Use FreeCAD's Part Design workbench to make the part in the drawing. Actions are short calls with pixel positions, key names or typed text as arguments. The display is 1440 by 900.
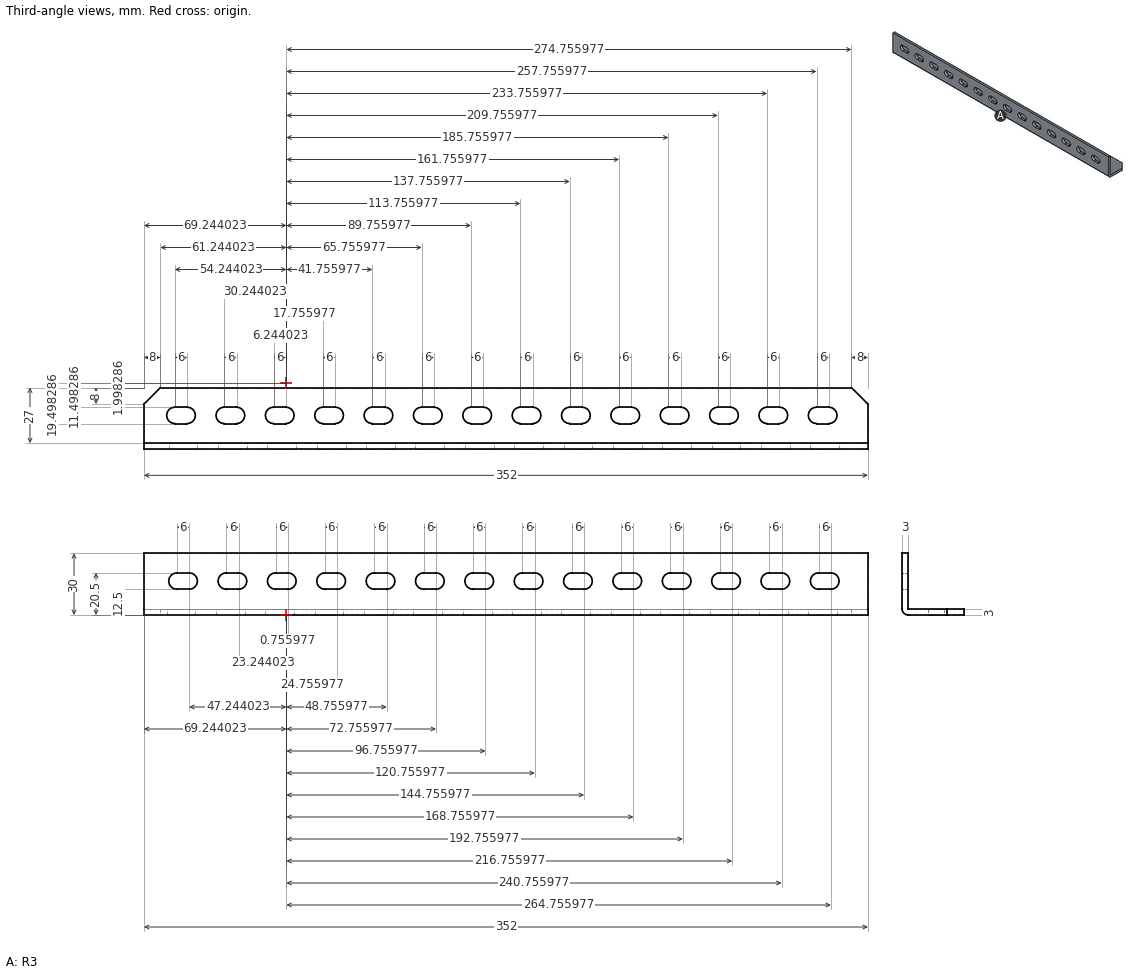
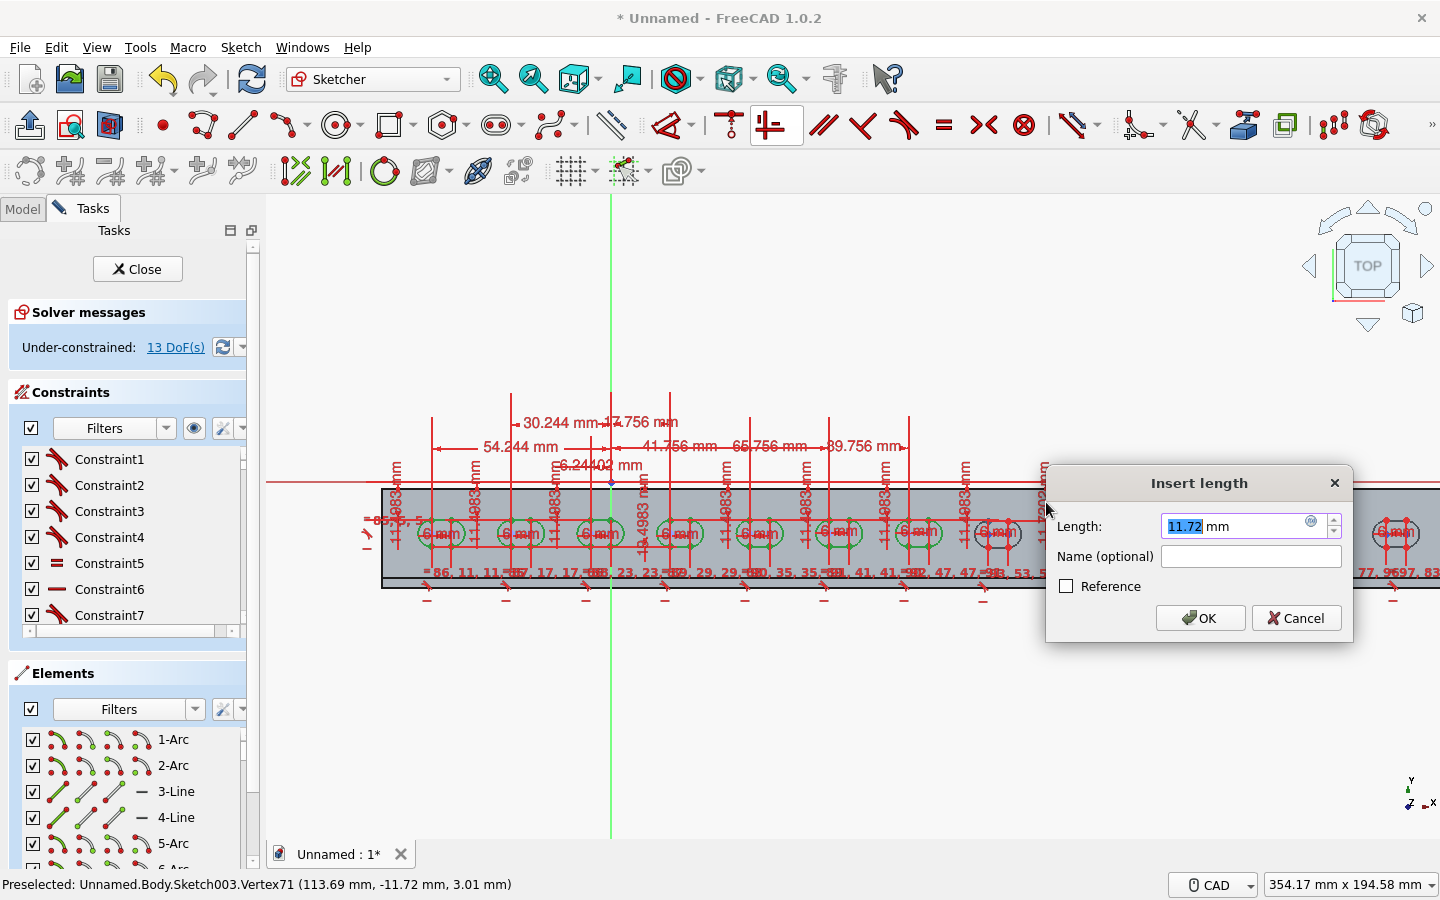
text(11.498286)
key(Return)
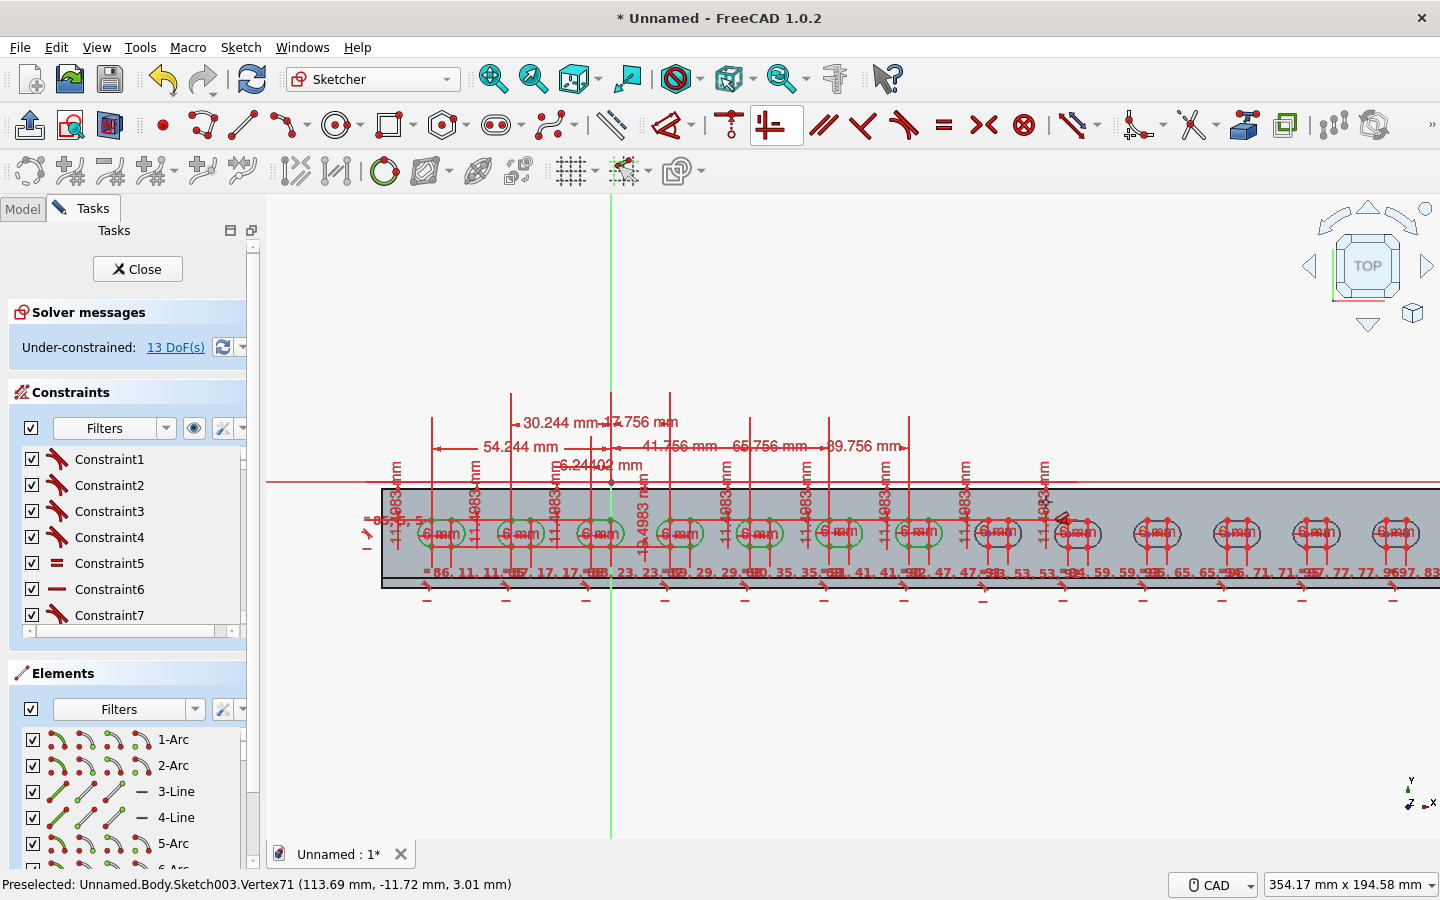
click(1068, 521)
click(1126, 502)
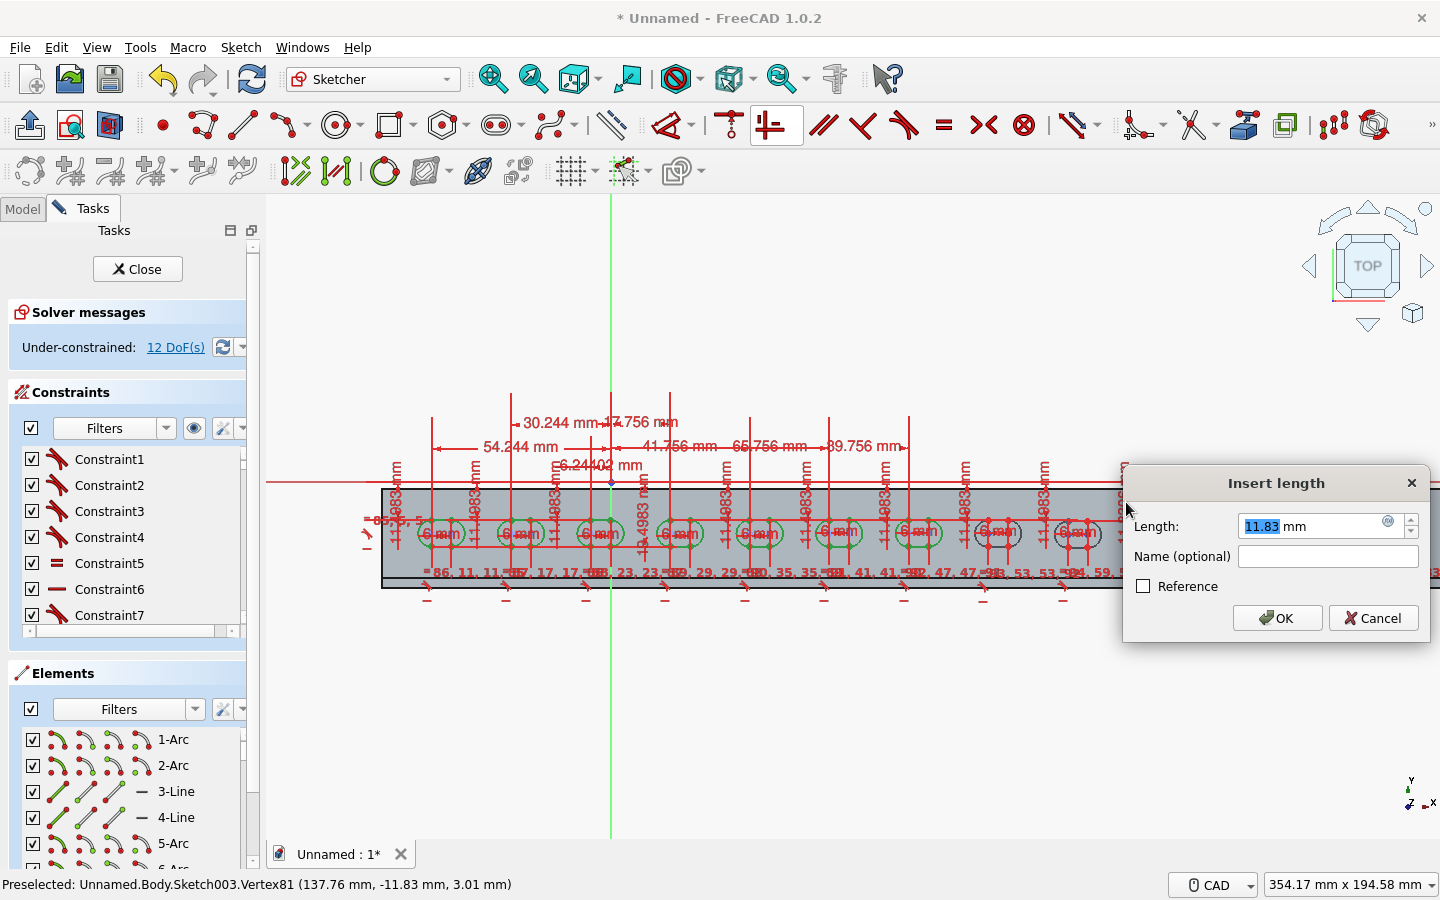
text(11.498286)
key(Return)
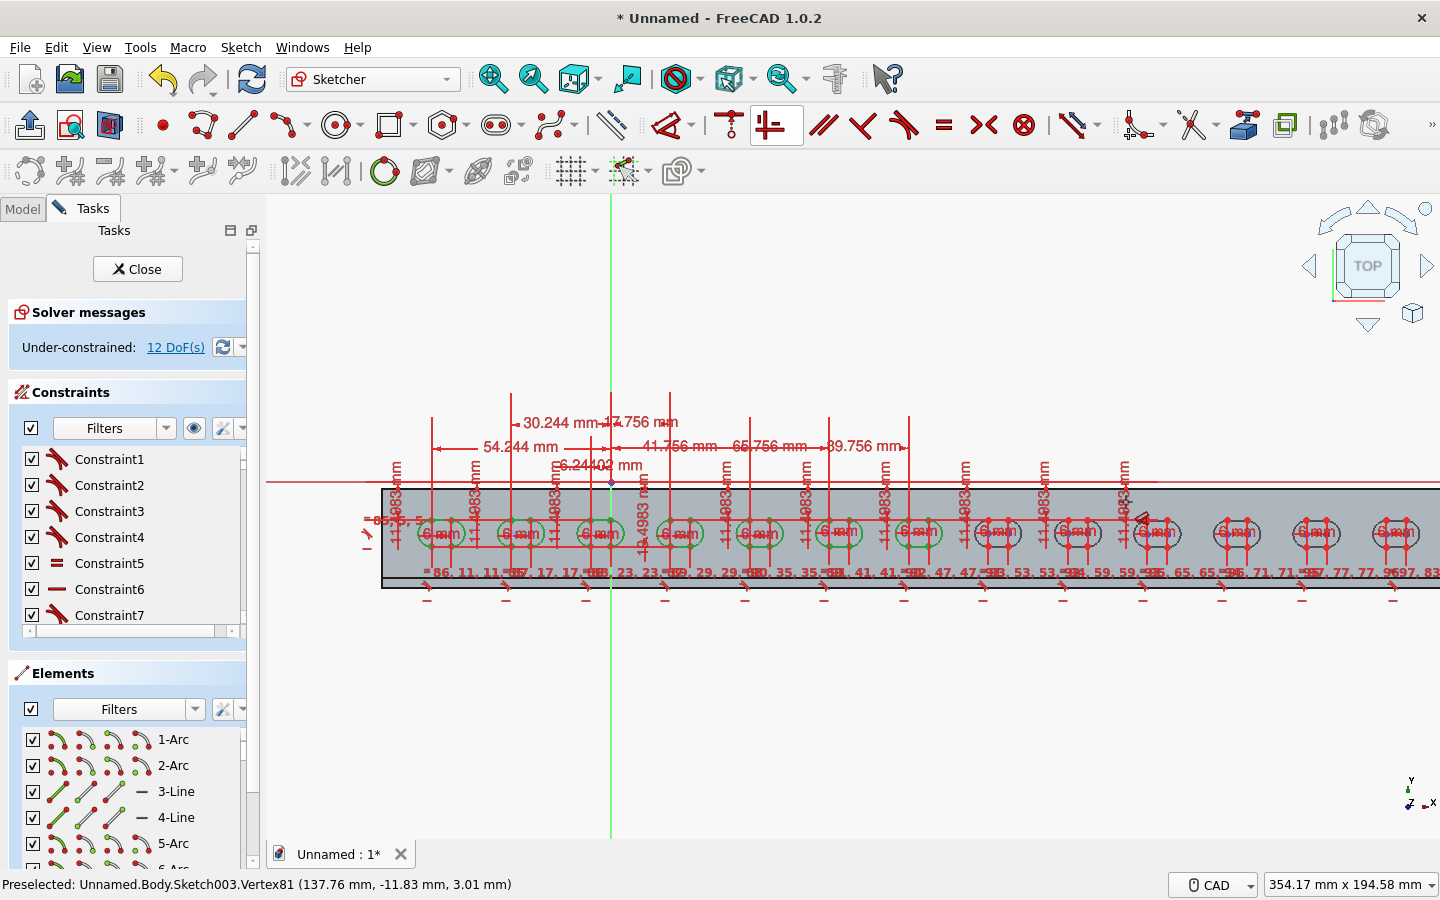
click(1147, 521)
click(1205, 502)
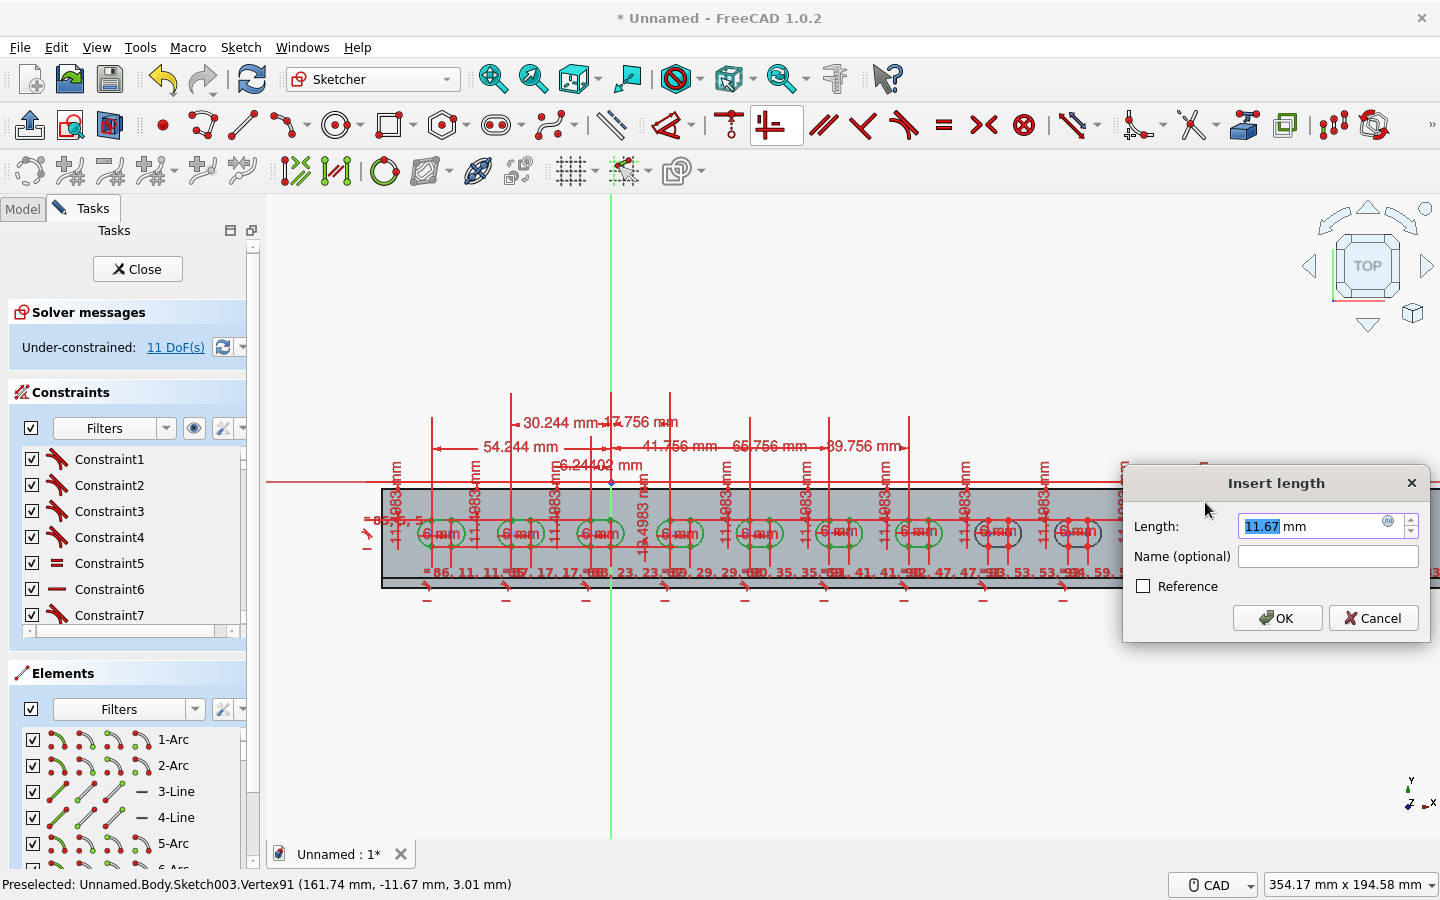
text(11.498286)
key(Return)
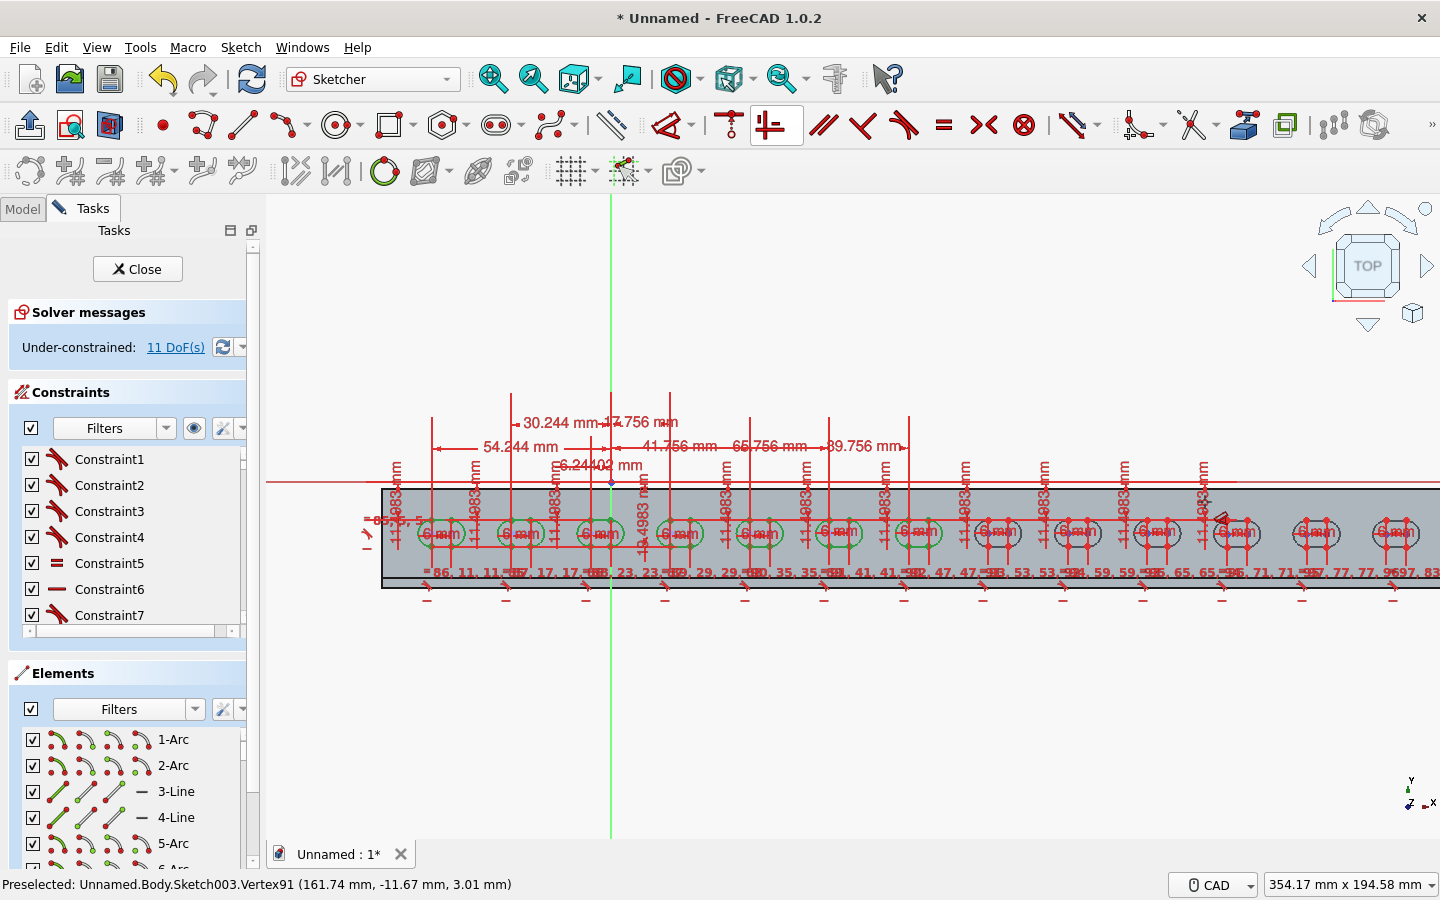
click(1227, 521)
click(577, 515)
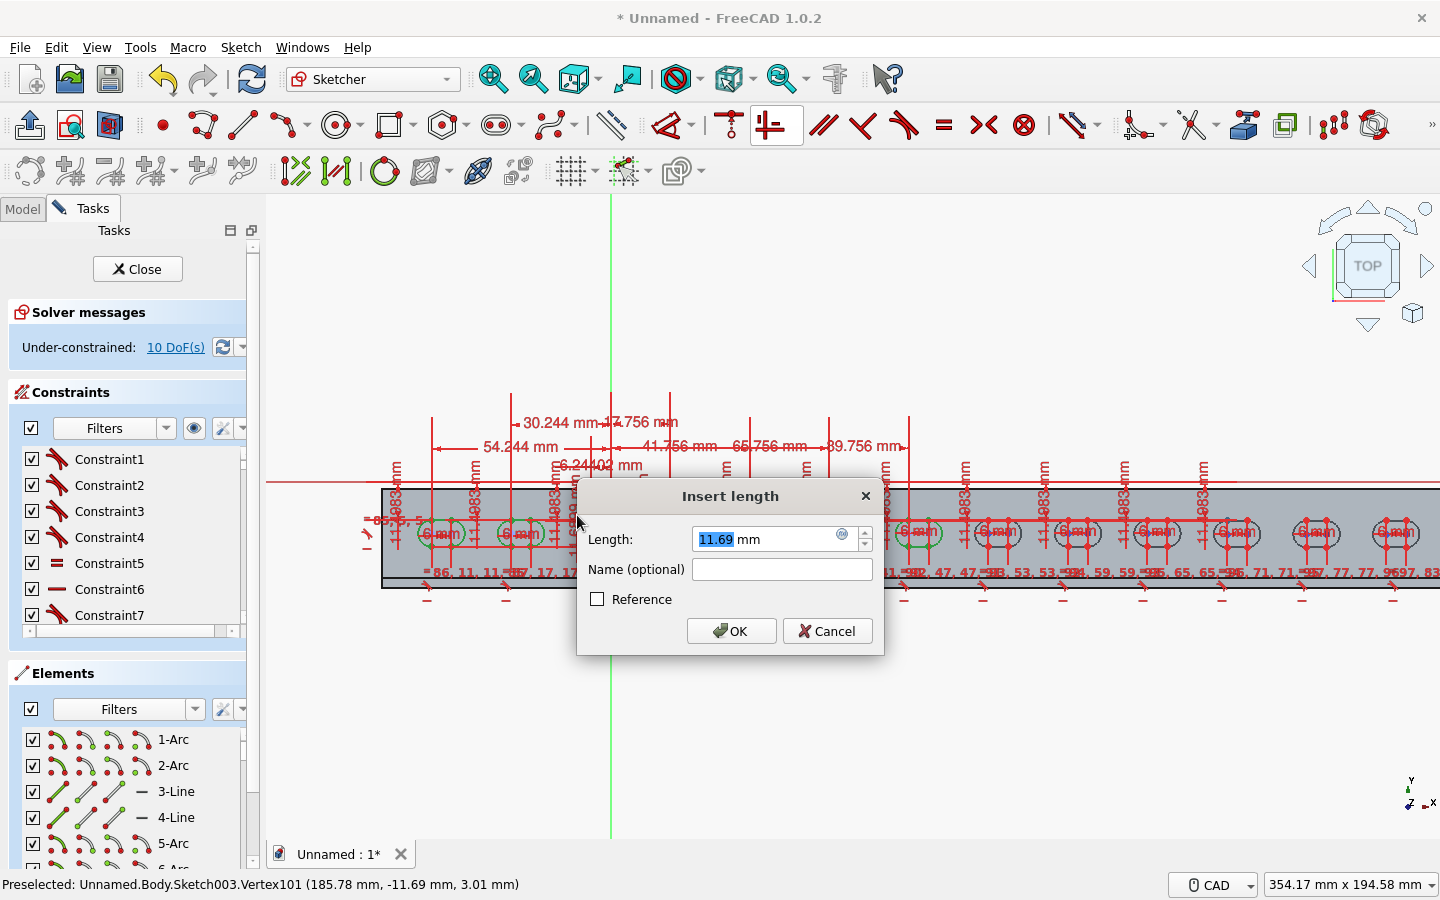
text(11.498286)
key(Return)